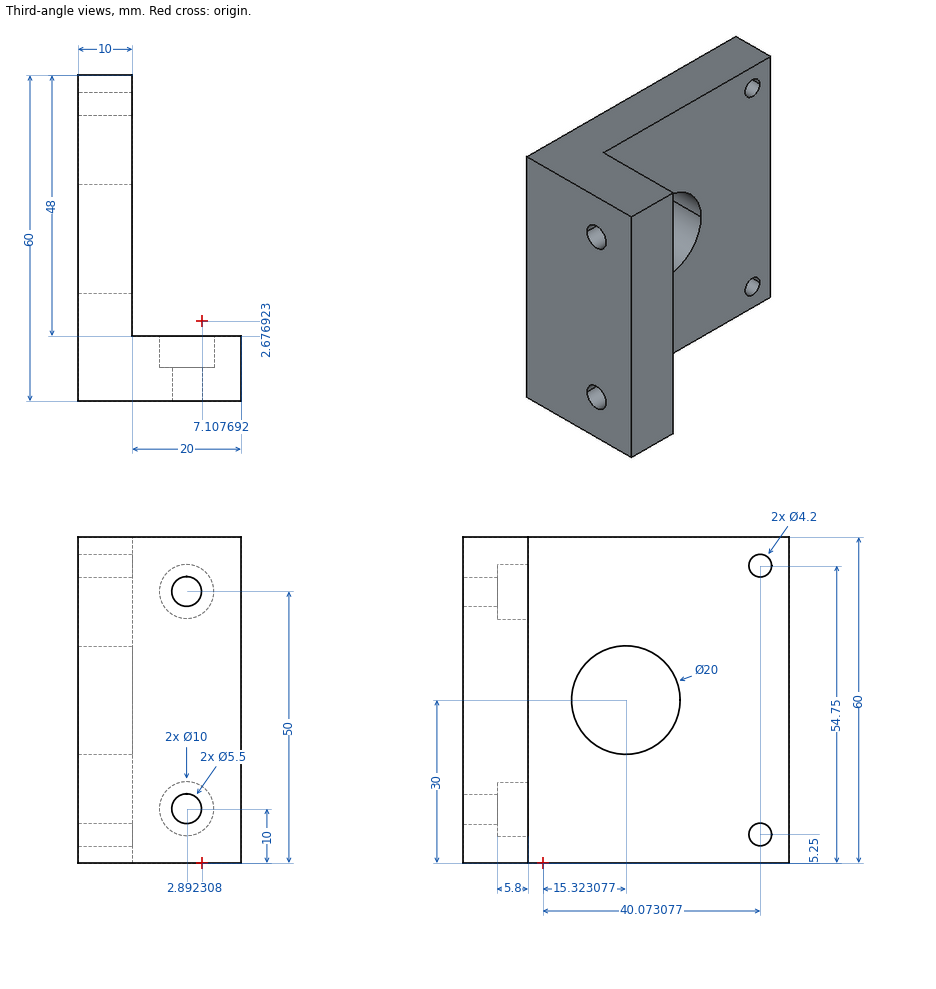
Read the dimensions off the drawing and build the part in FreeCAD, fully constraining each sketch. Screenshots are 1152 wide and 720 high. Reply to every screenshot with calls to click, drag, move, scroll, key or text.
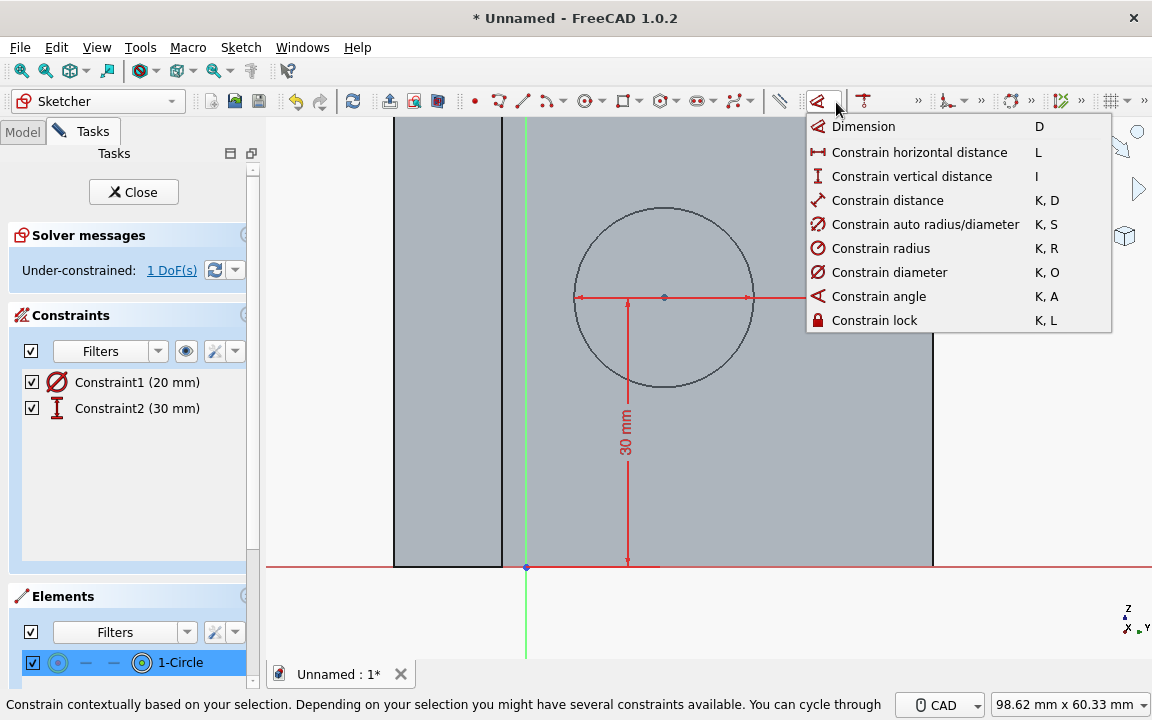
click(959, 152)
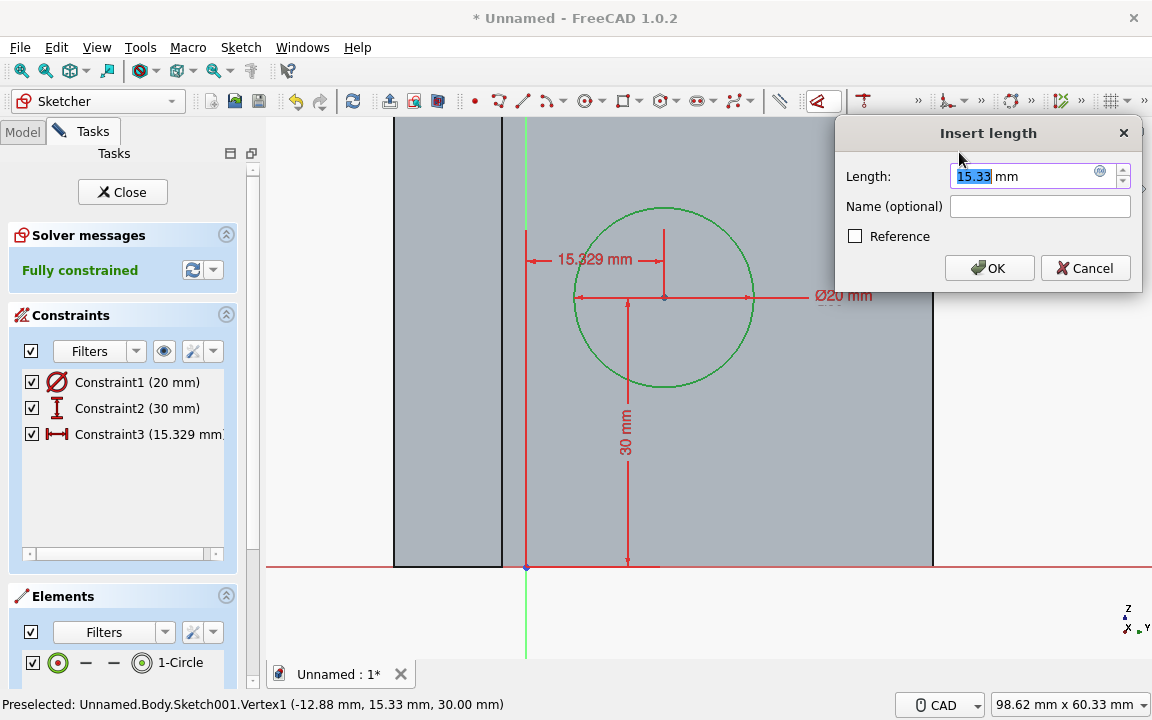
text(15.323077)
key(Return)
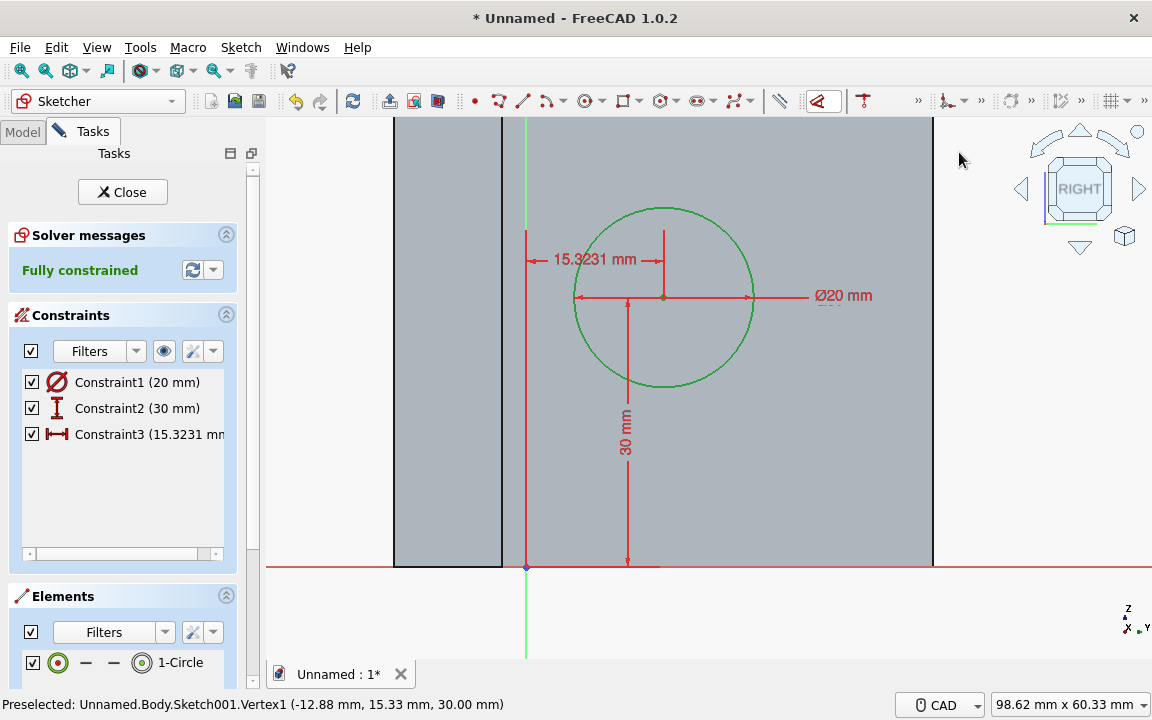
click(123, 192)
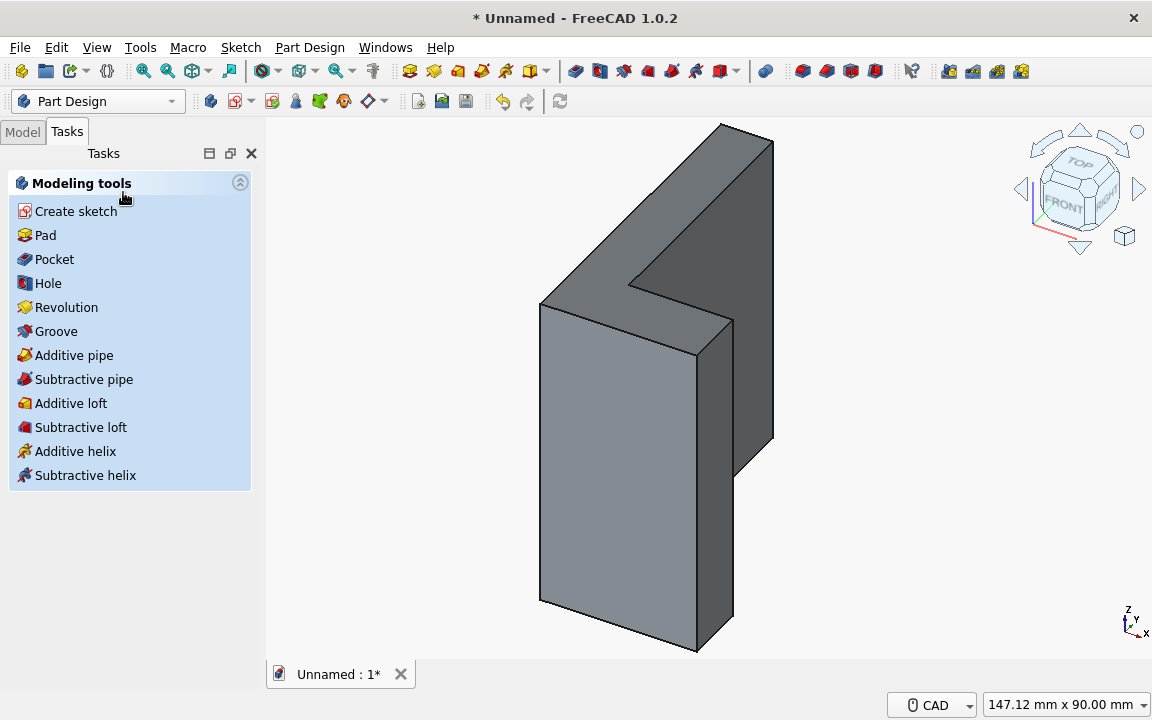
click(576, 72)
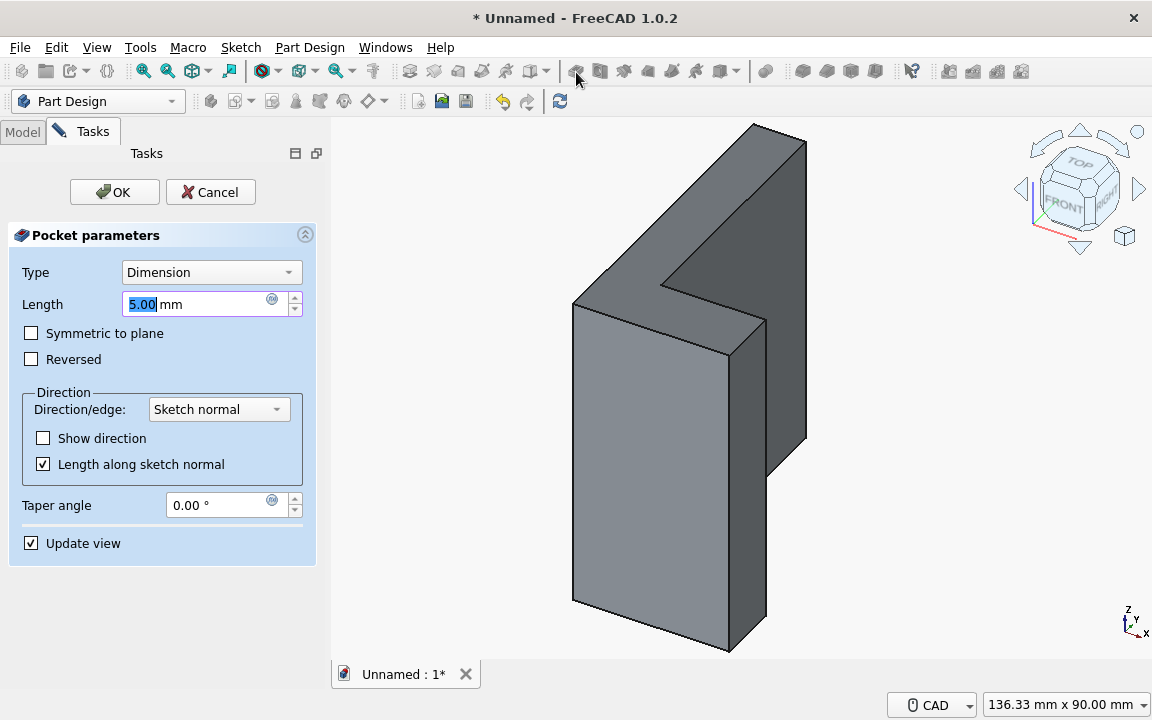
click(212, 272)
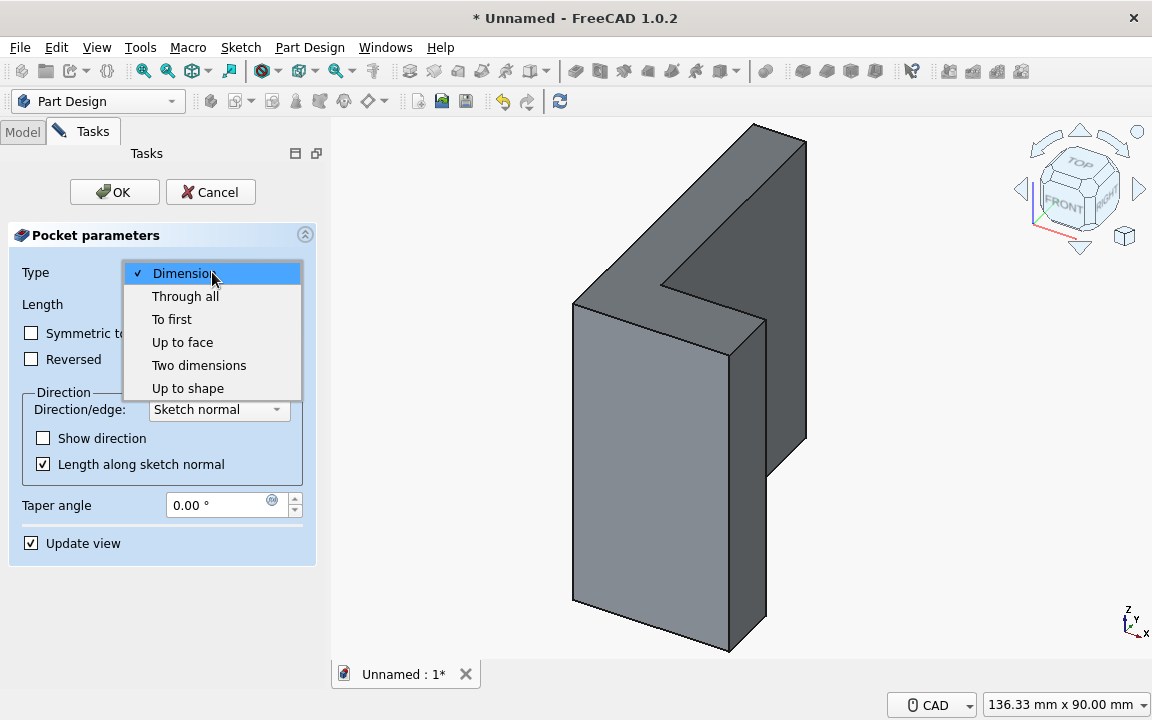
click(212, 296)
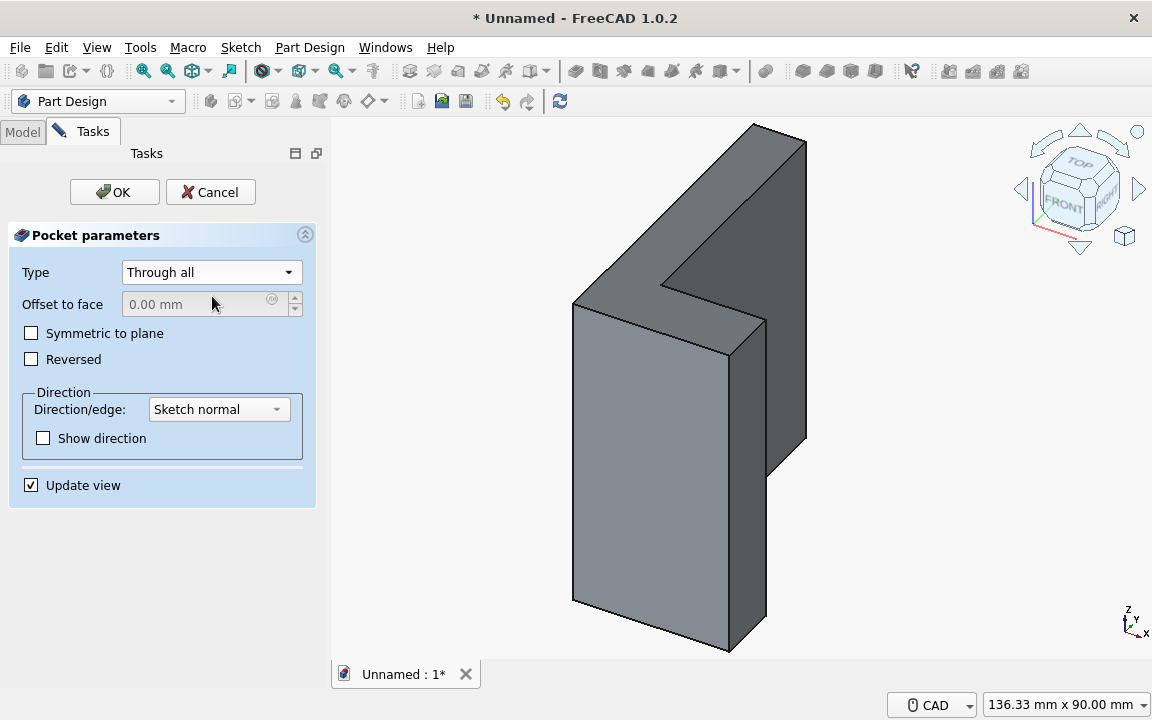
click(115, 192)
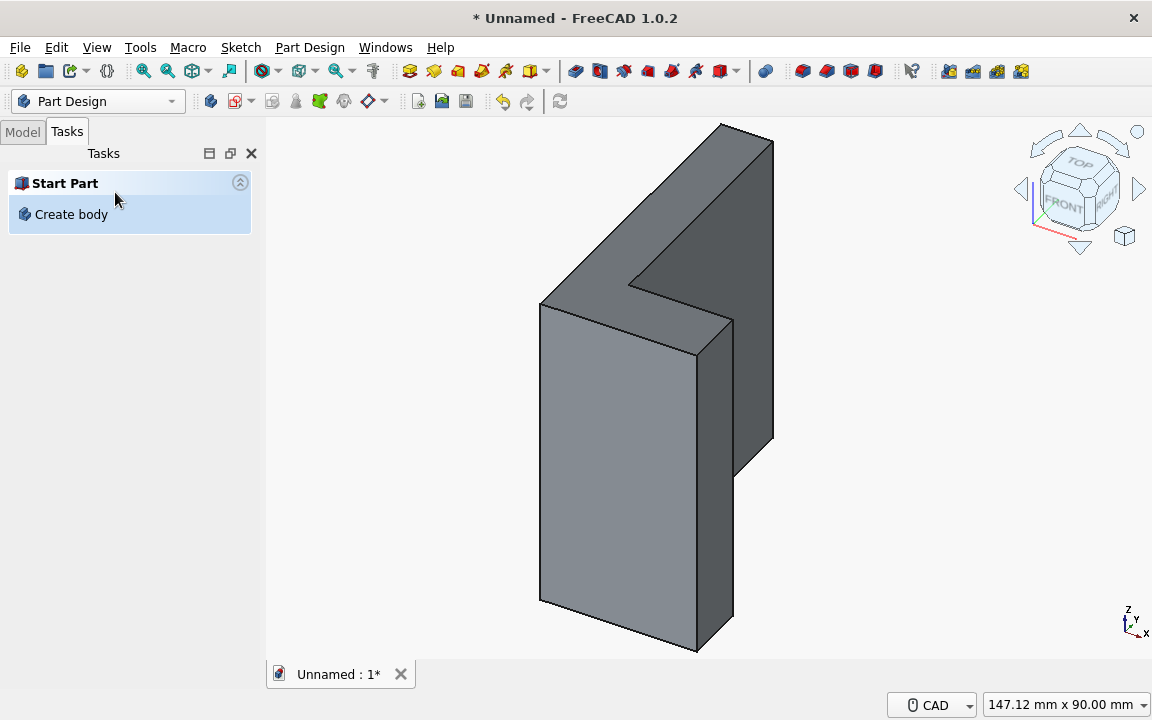
click(722, 255)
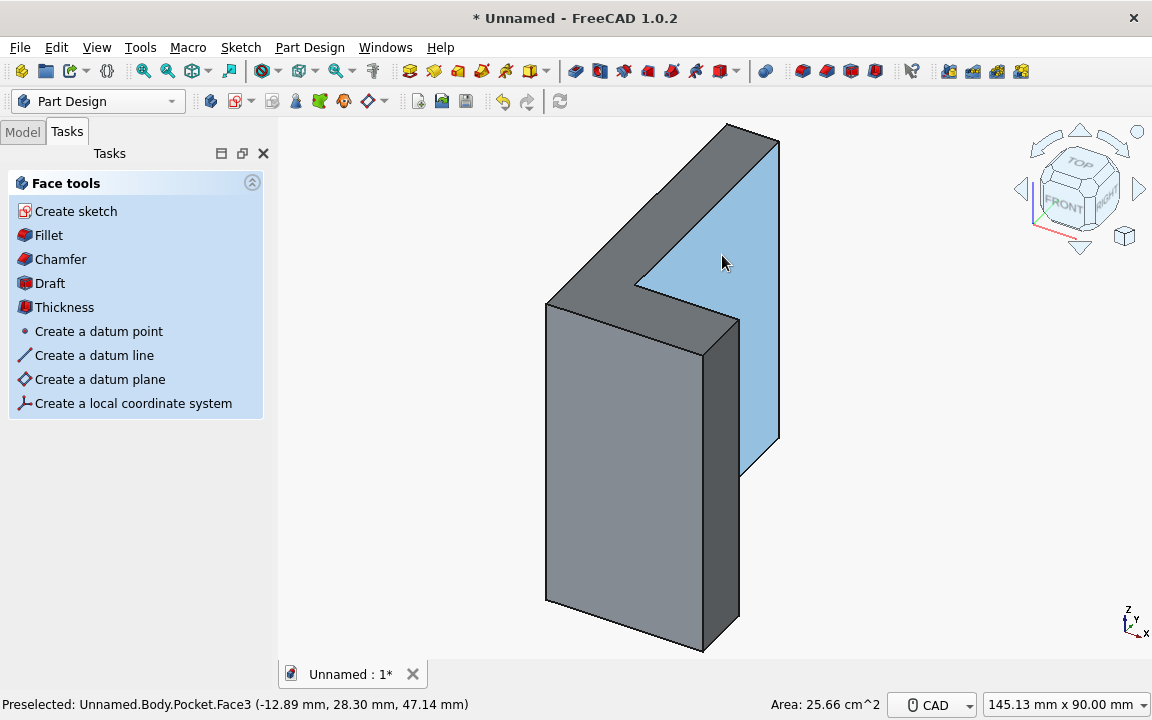
click(236, 102)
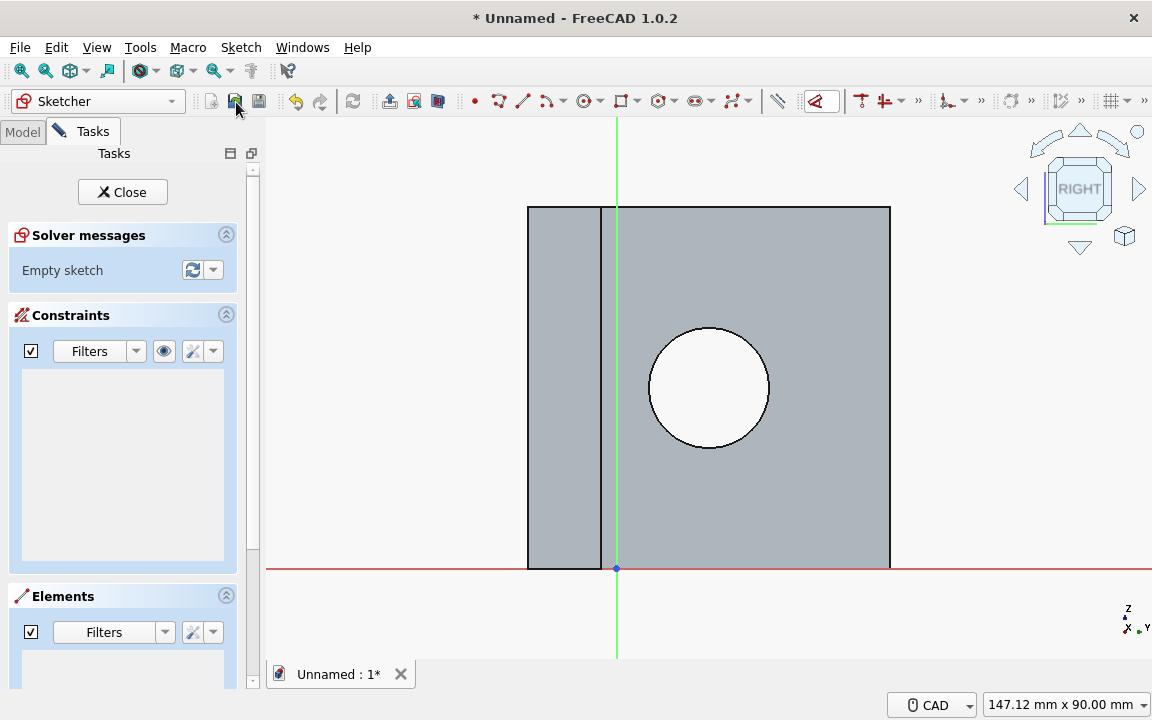
click(584, 102)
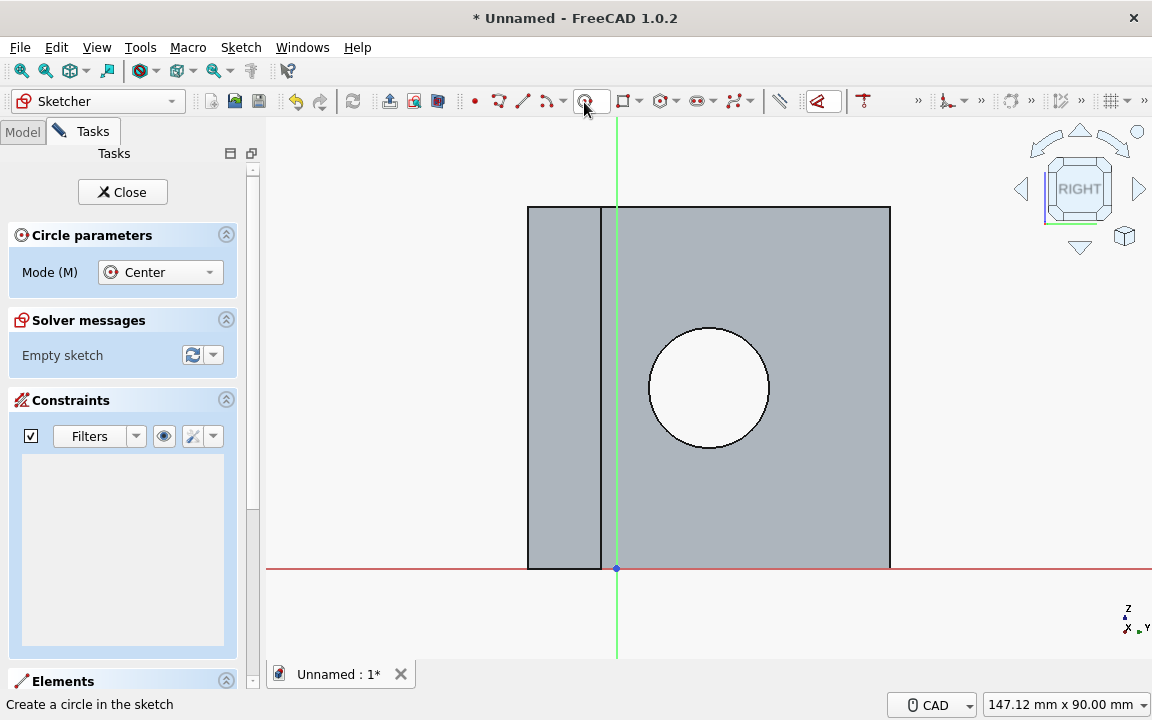
scroll(858, 239, up, 3)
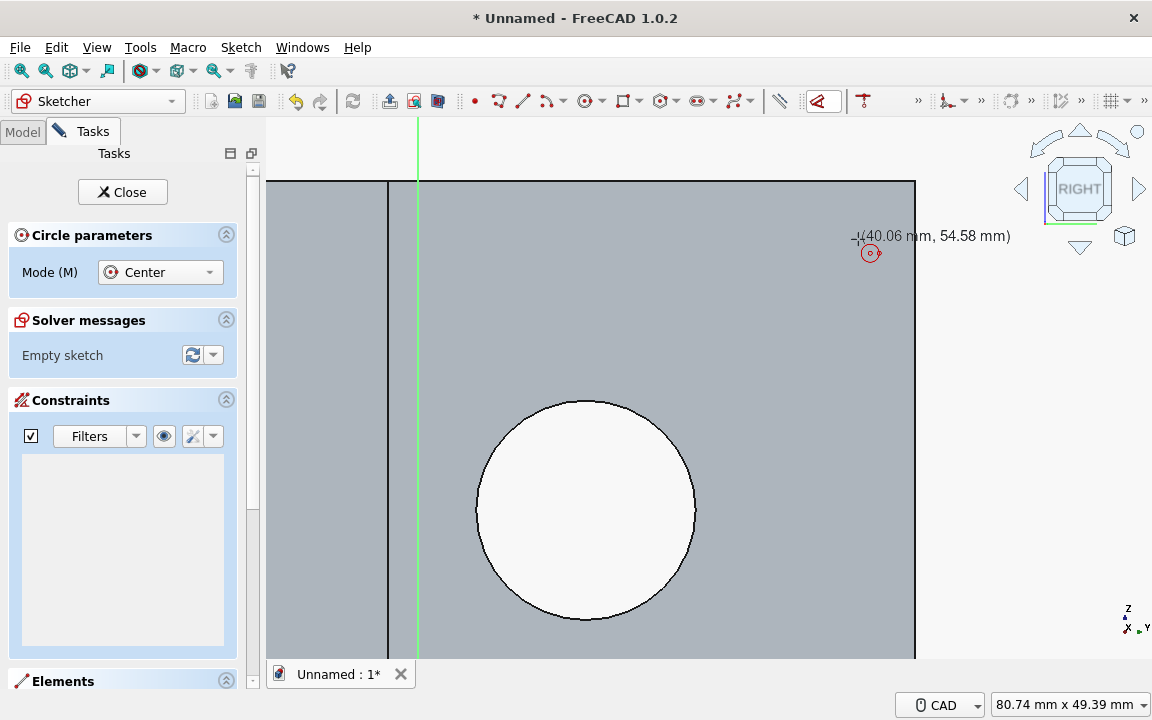
click(858, 239)
move(874, 222)